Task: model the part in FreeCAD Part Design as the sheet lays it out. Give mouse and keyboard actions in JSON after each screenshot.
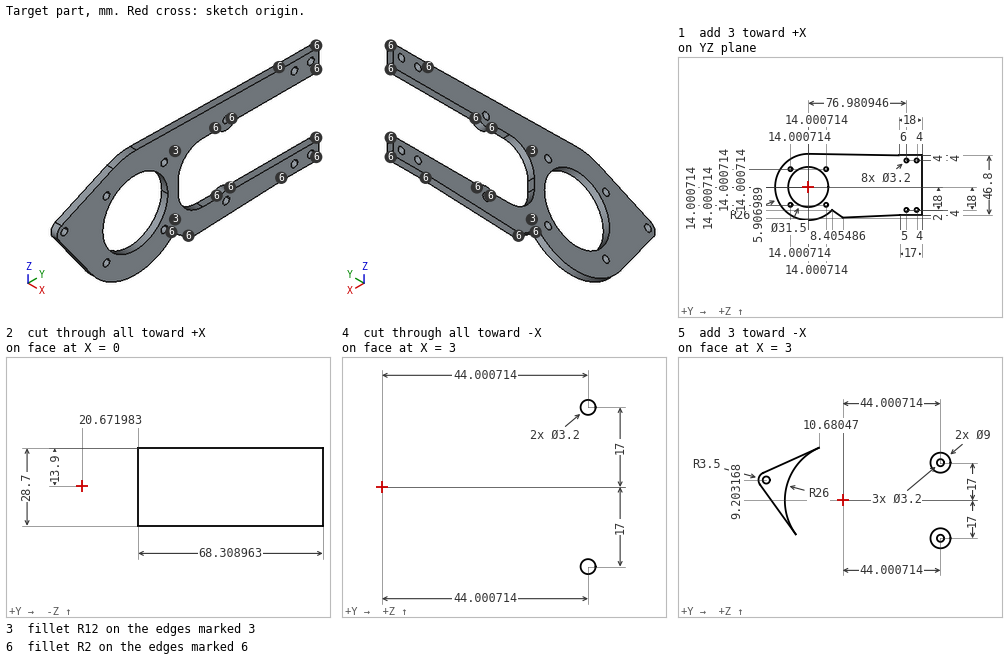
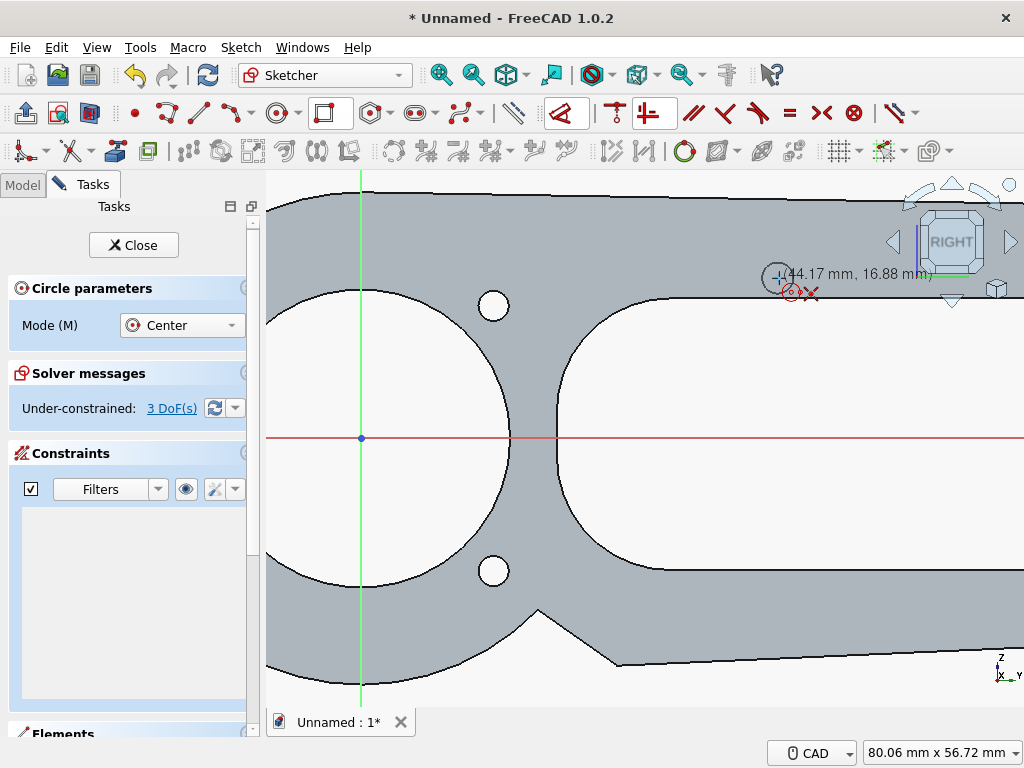
{"action": "scroll", "coordinate": [778, 599], "scroll_direction": "up", "scroll_amount": 3}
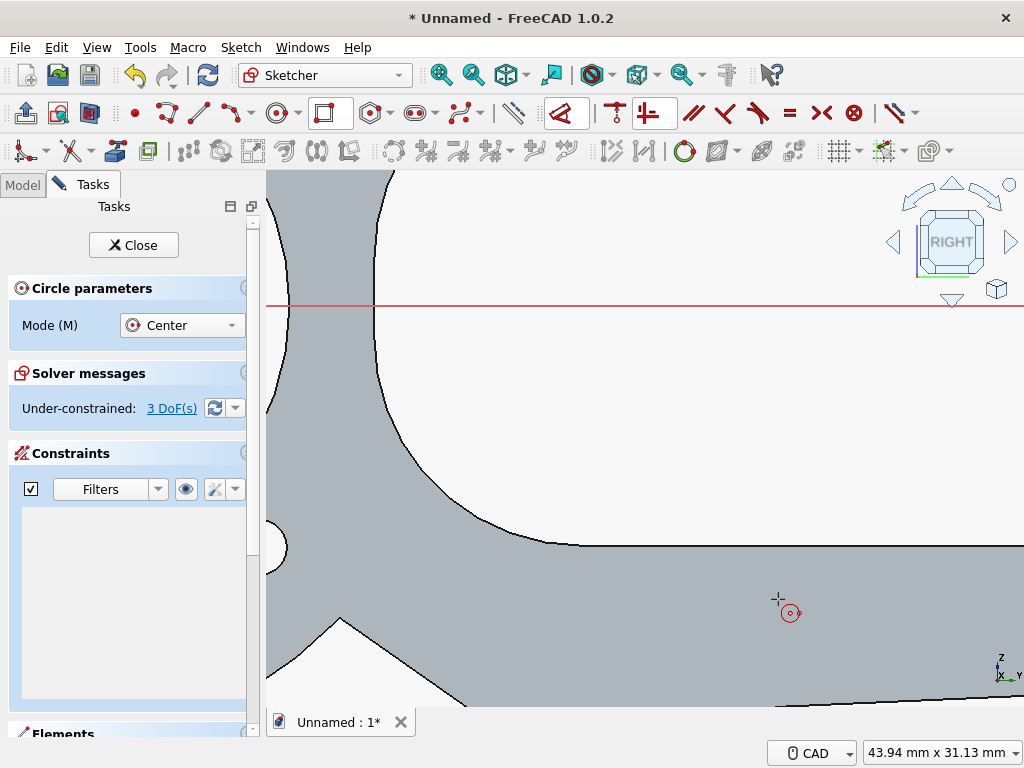
{"action": "left_click", "coordinate": [777, 599]}
{"action": "left_click", "coordinate": [796, 580]}
{"action": "key", "text": "Escape"}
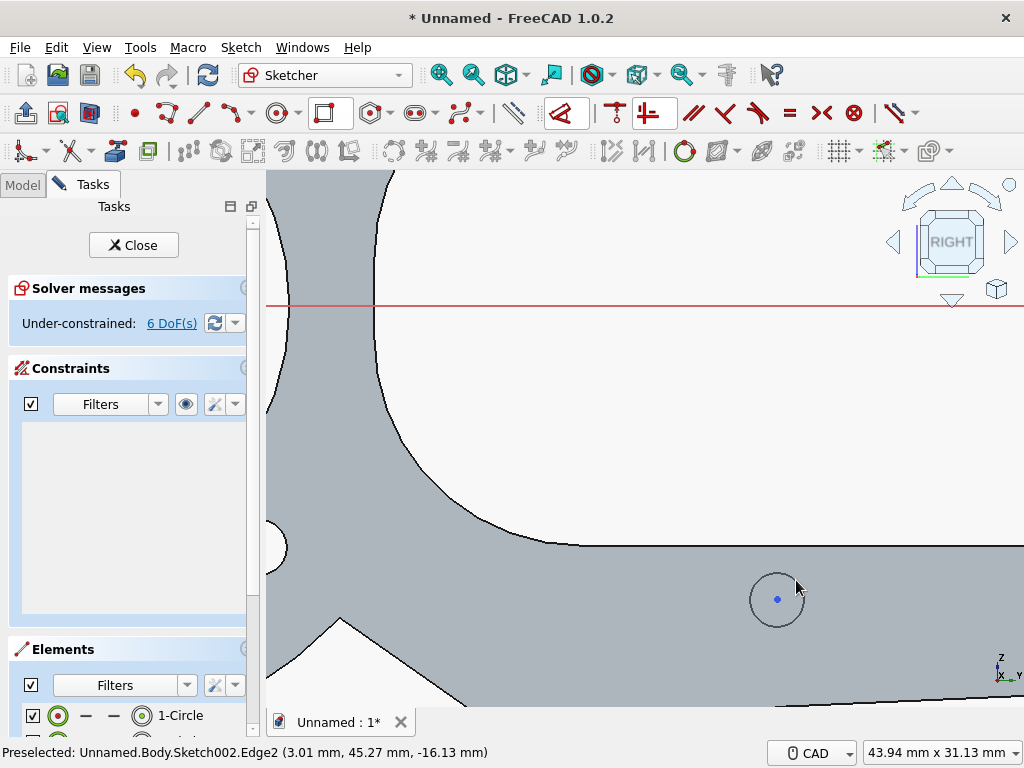
{"action": "scroll", "coordinate": [778, 600], "scroll_direction": "down", "scroll_amount": 3}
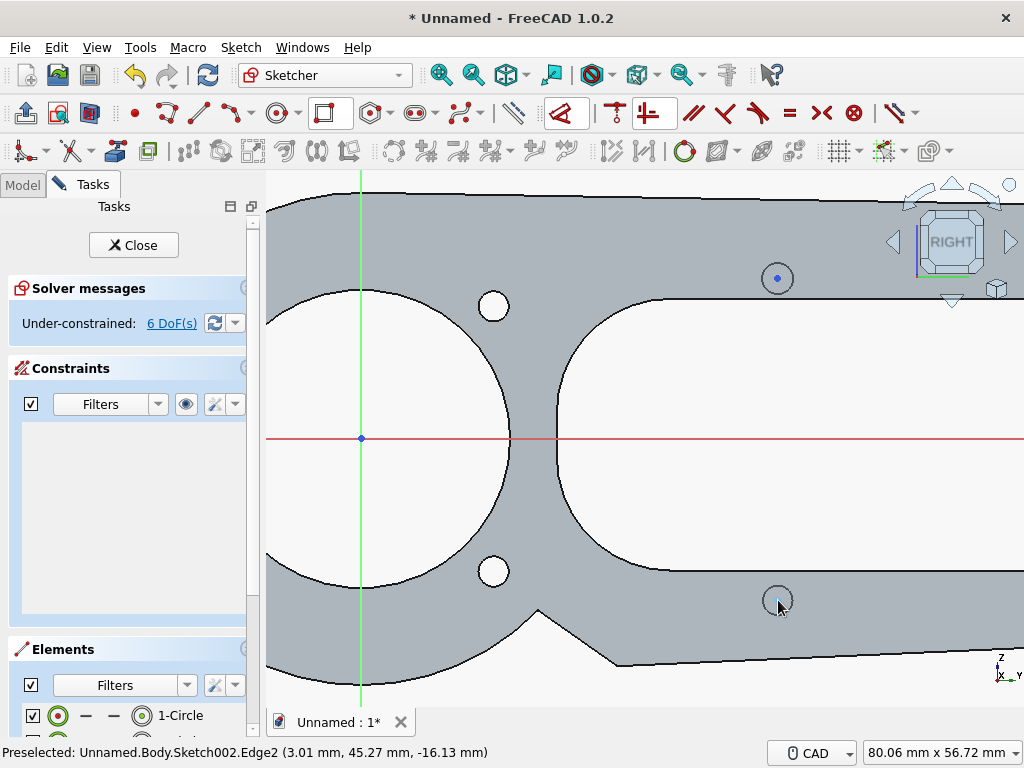
{"action": "left_click", "coordinate": [789, 268]}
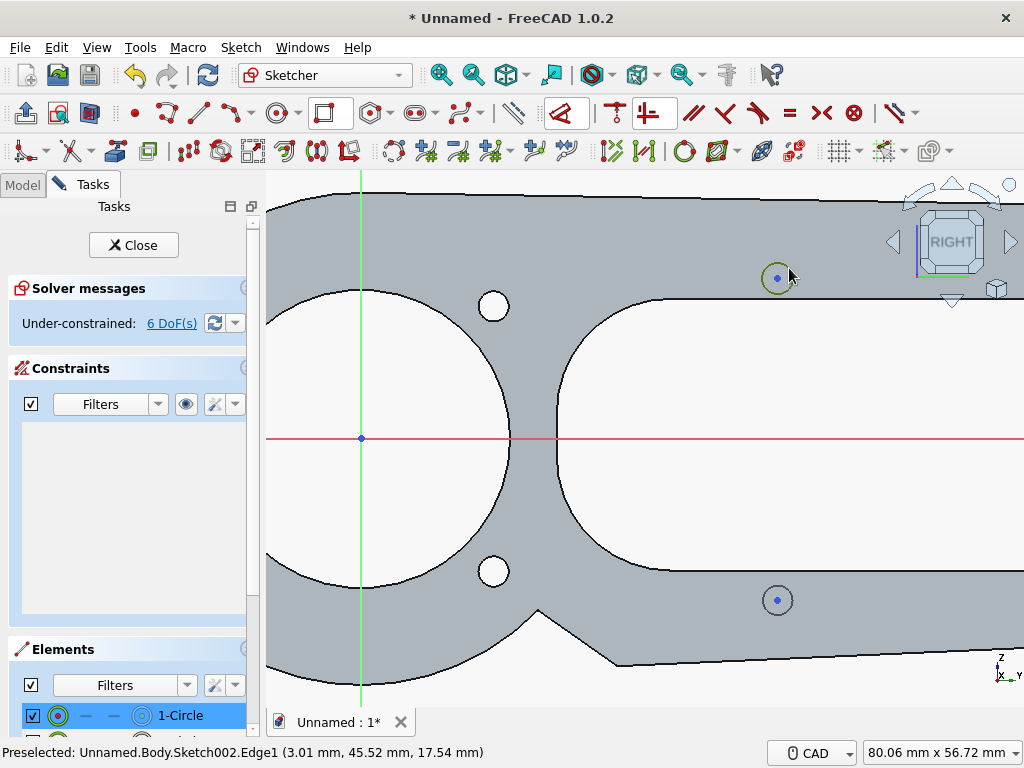
{"action": "left_click", "coordinate": [788, 590]}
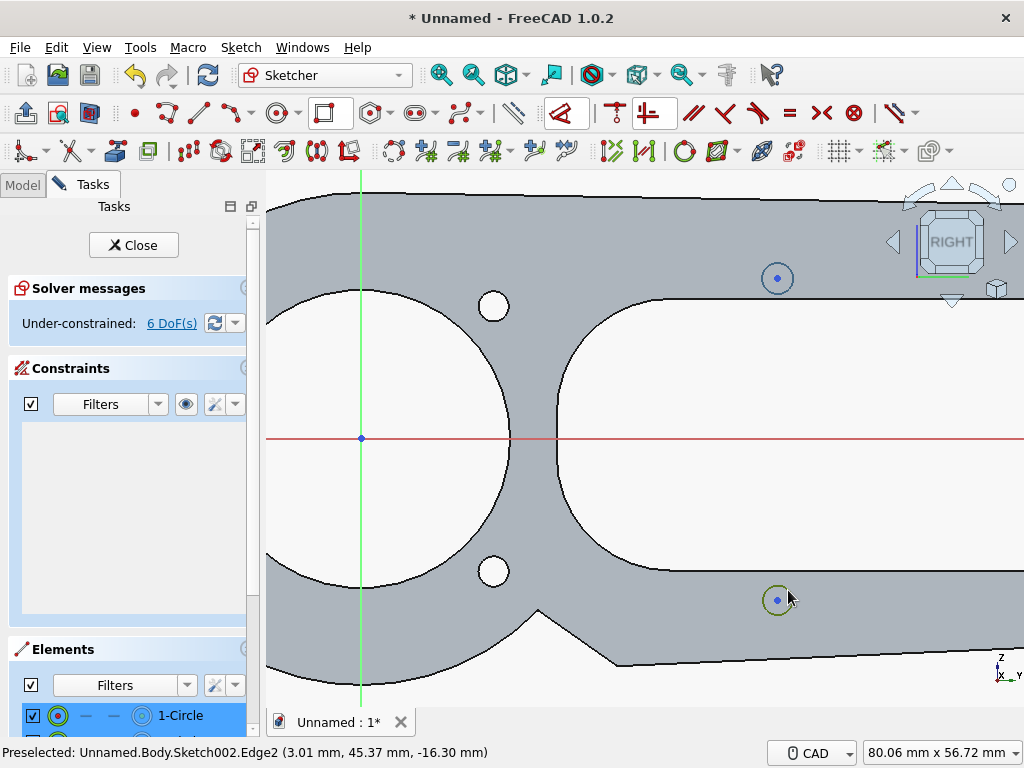
{"action": "left_click", "coordinate": [790, 114]}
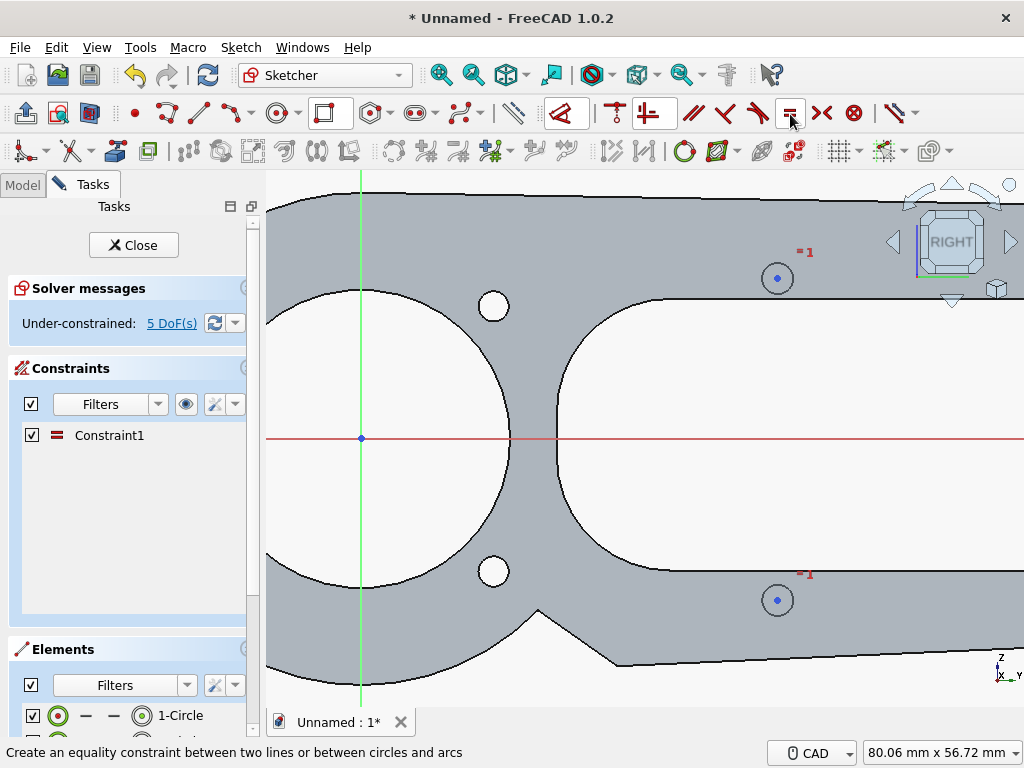
{"action": "scroll", "coordinate": [789, 268], "scroll_direction": "up", "scroll_amount": 2}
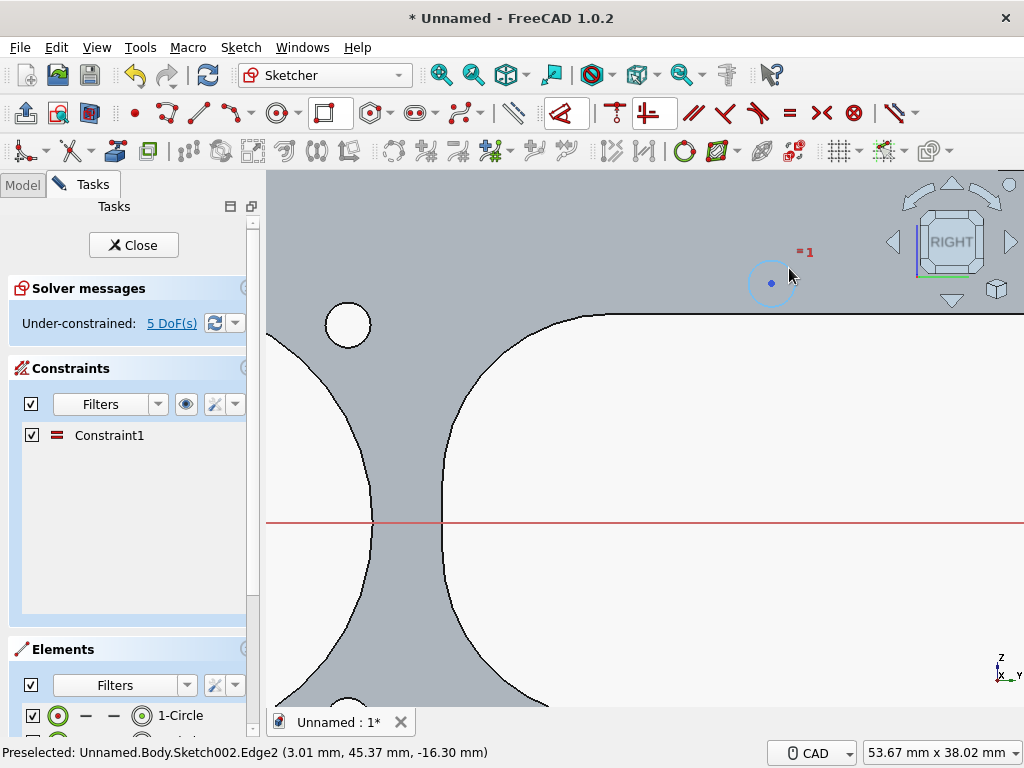
{"action": "left_click", "coordinate": [788, 267]}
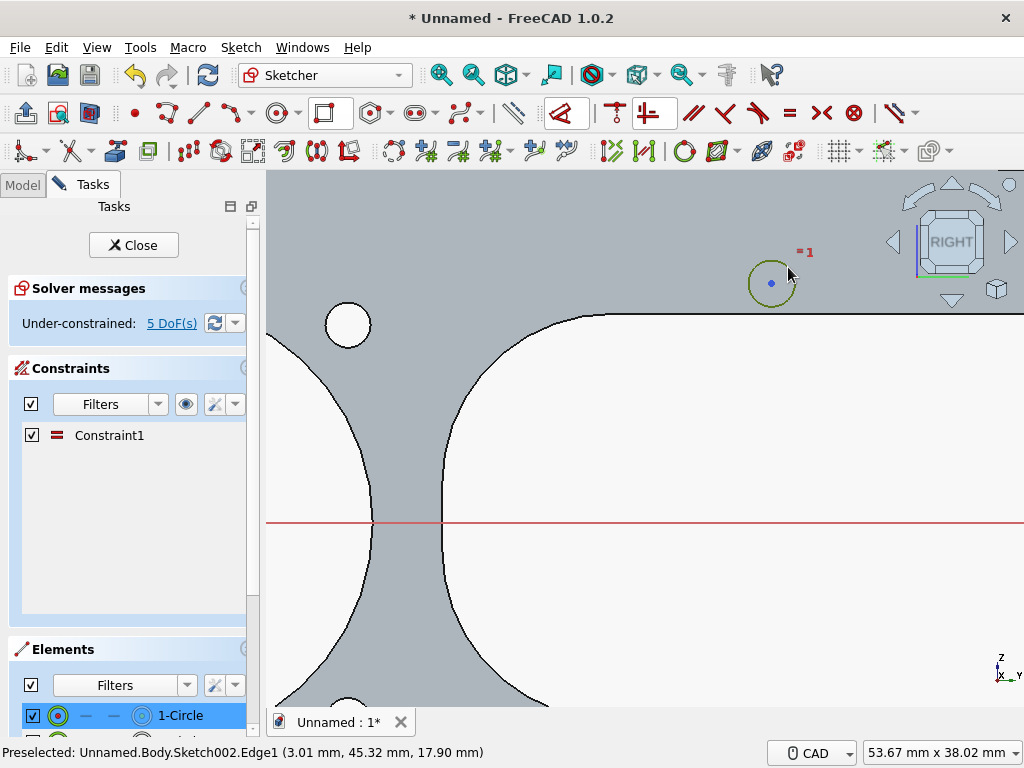
{"action": "left_click", "coordinate": [584, 114]}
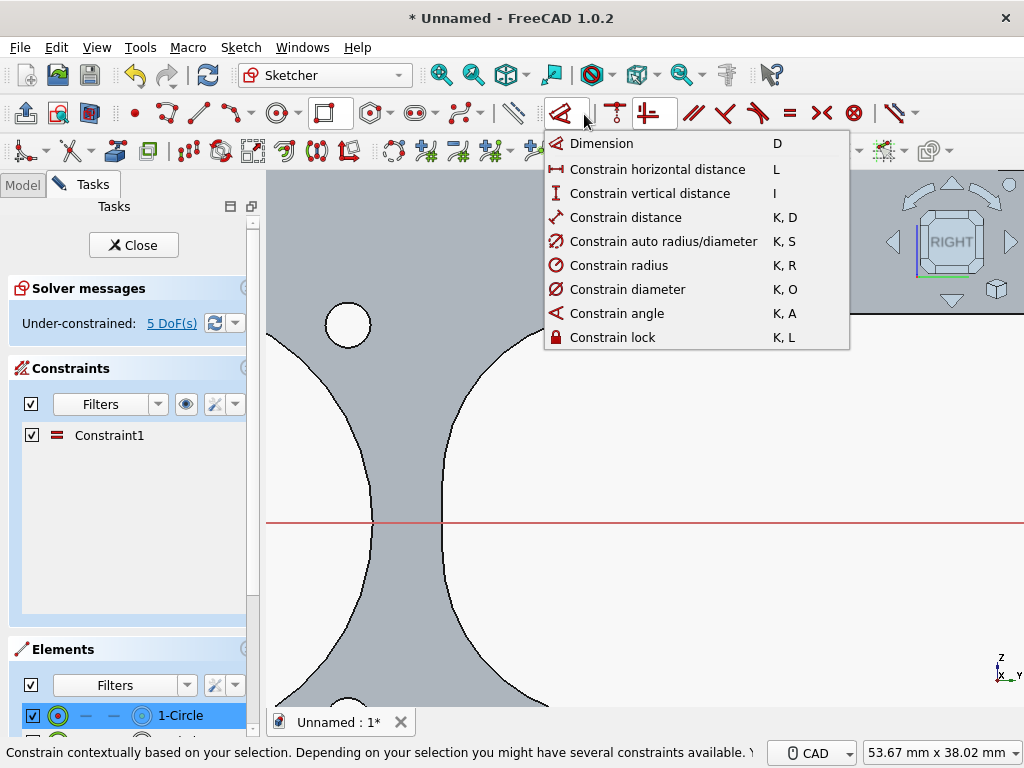
{"action": "left_click", "coordinate": [697, 289]}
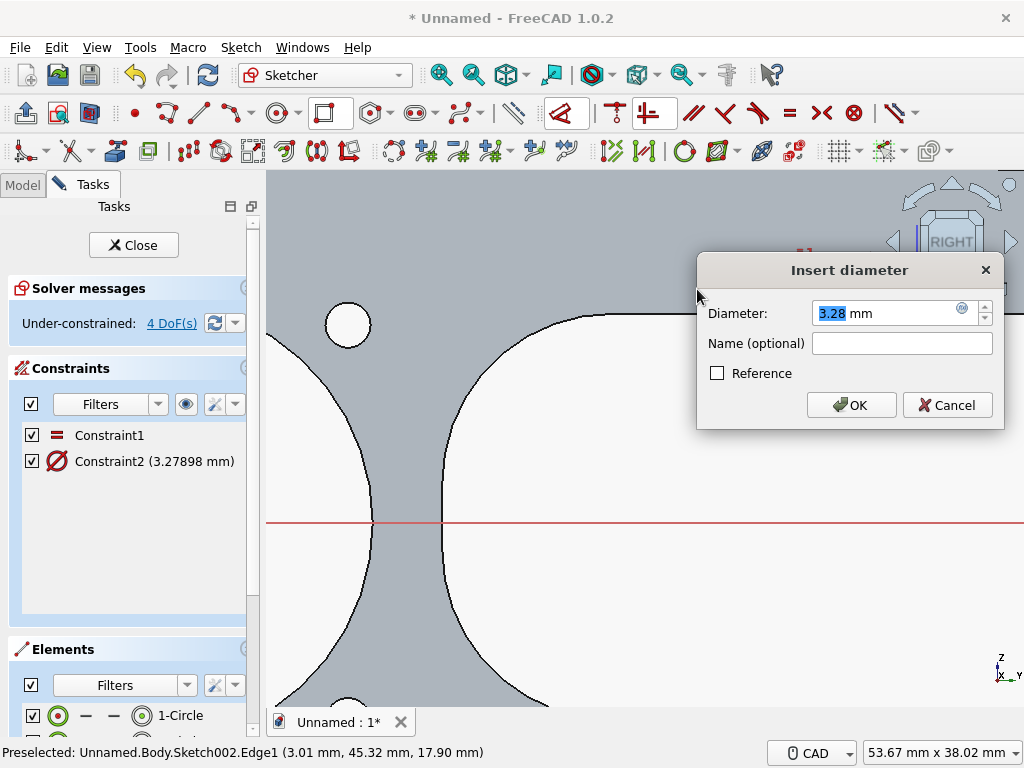
{"action": "type", "text": "3.2"}
{"action": "key", "text": "Return"}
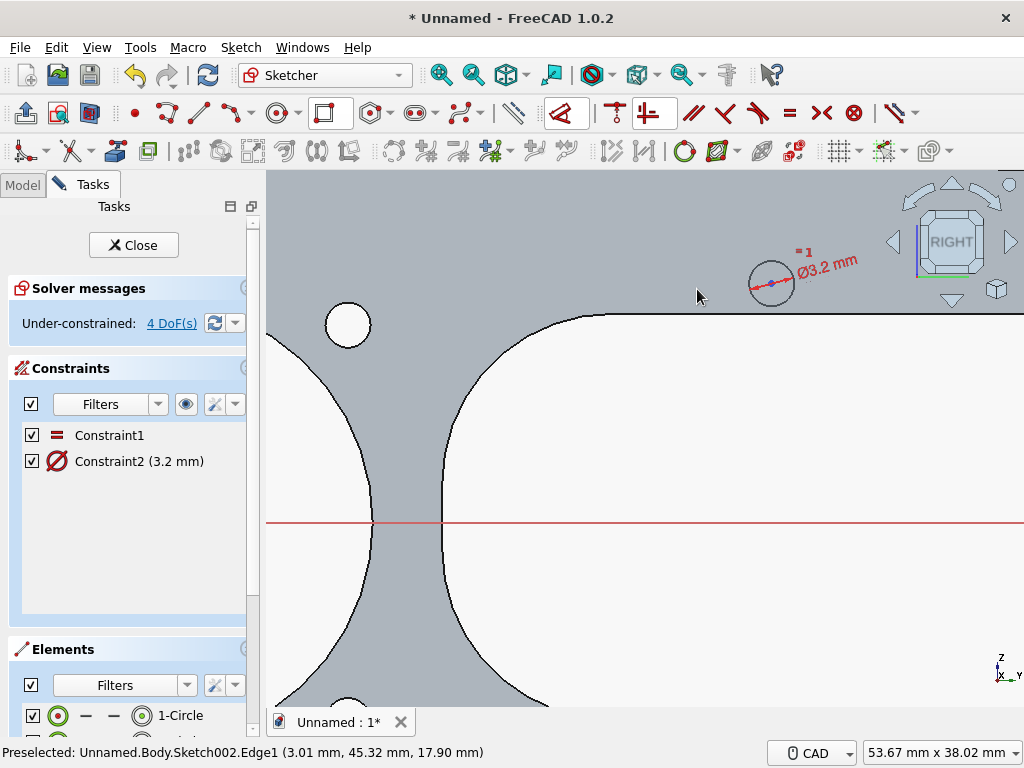
{"action": "left_click", "coordinate": [772, 284]}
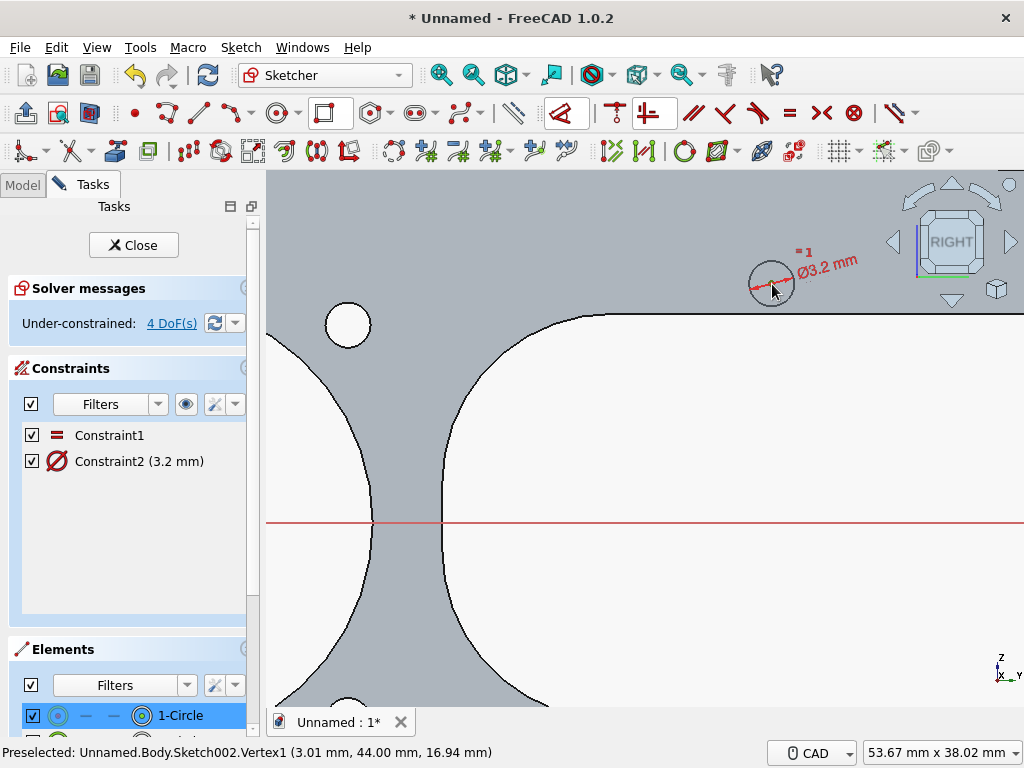
{"action": "key", "text": "i"}